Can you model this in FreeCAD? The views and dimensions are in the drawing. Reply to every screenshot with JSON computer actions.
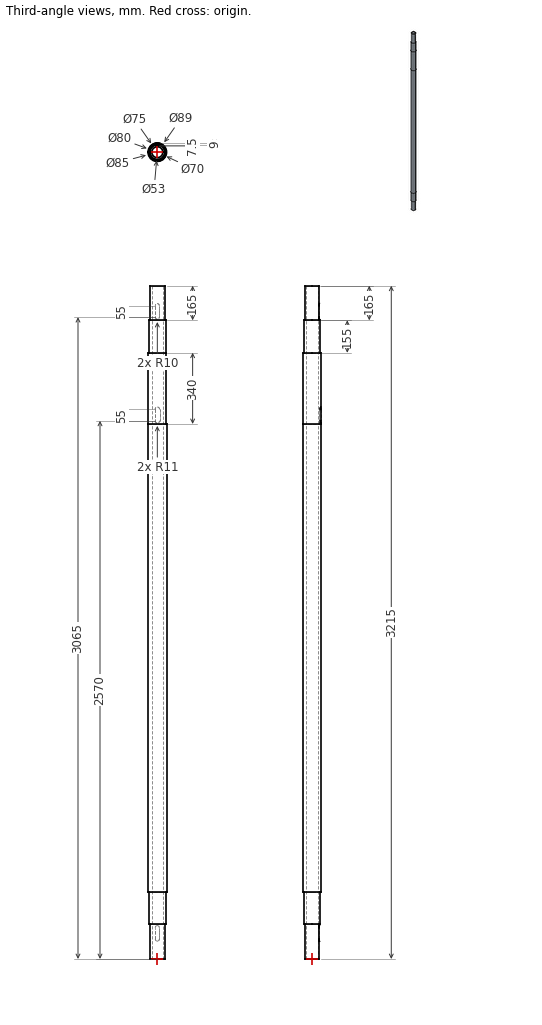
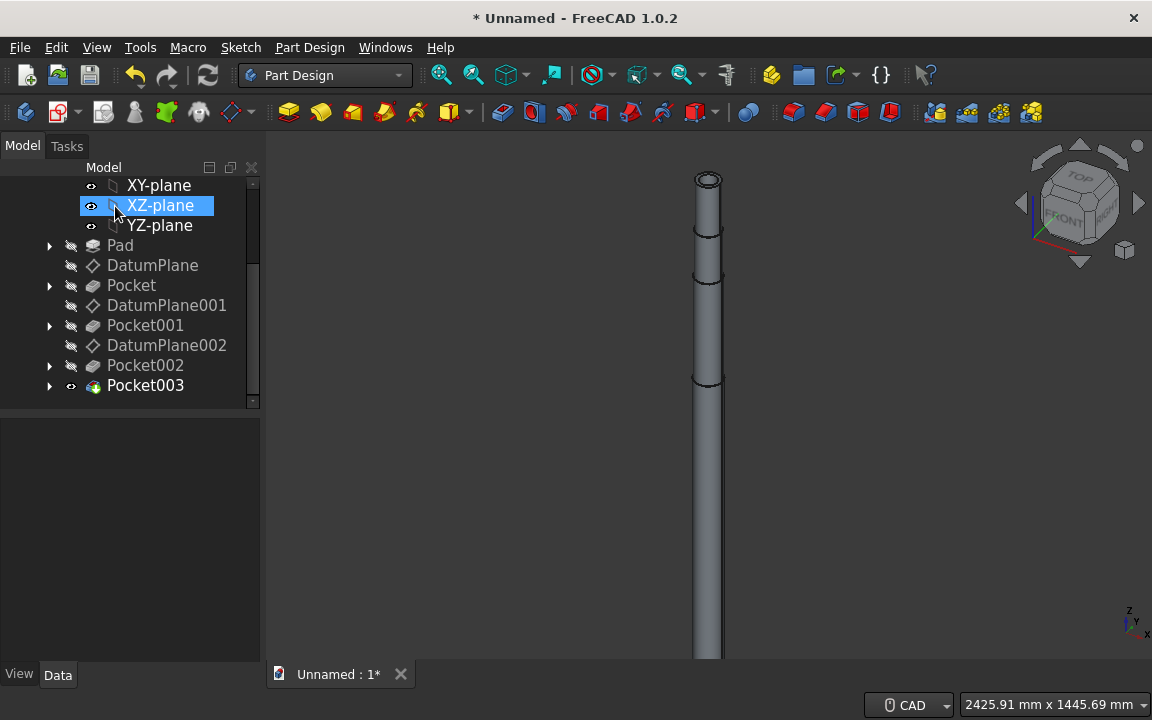
{"action": "left_click", "coordinate": [442, 76]}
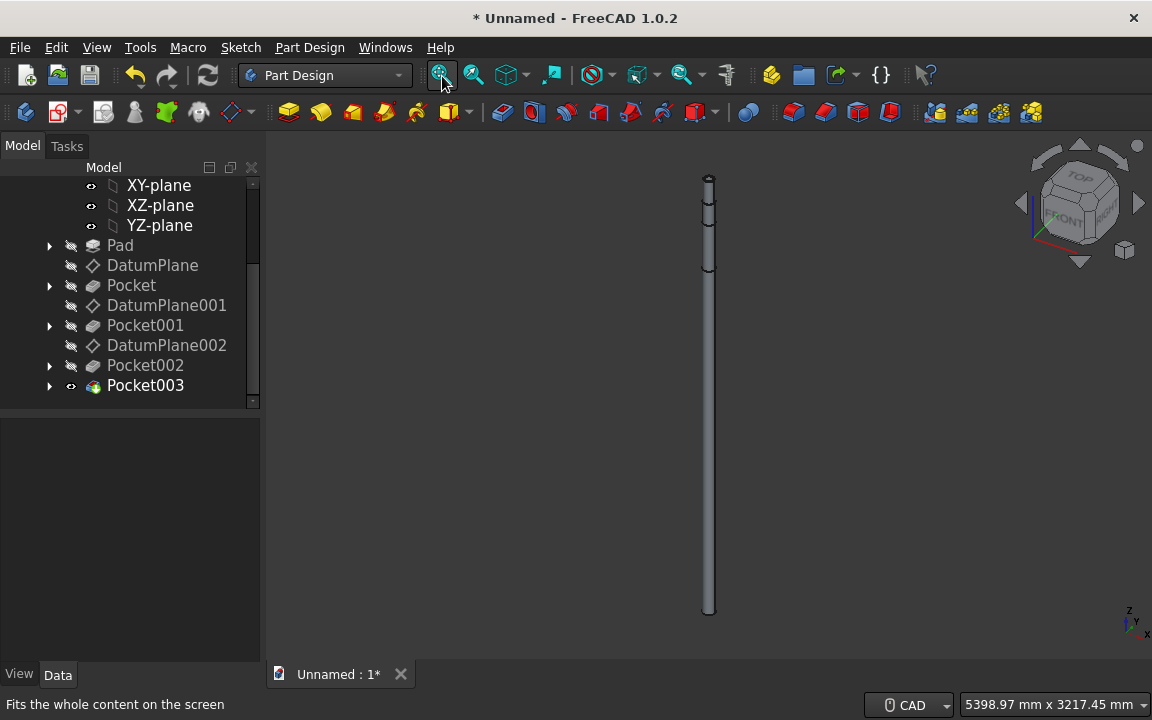
{"action": "scroll", "coordinate": [711, 197], "scroll_direction": "up", "scroll_amount": 15}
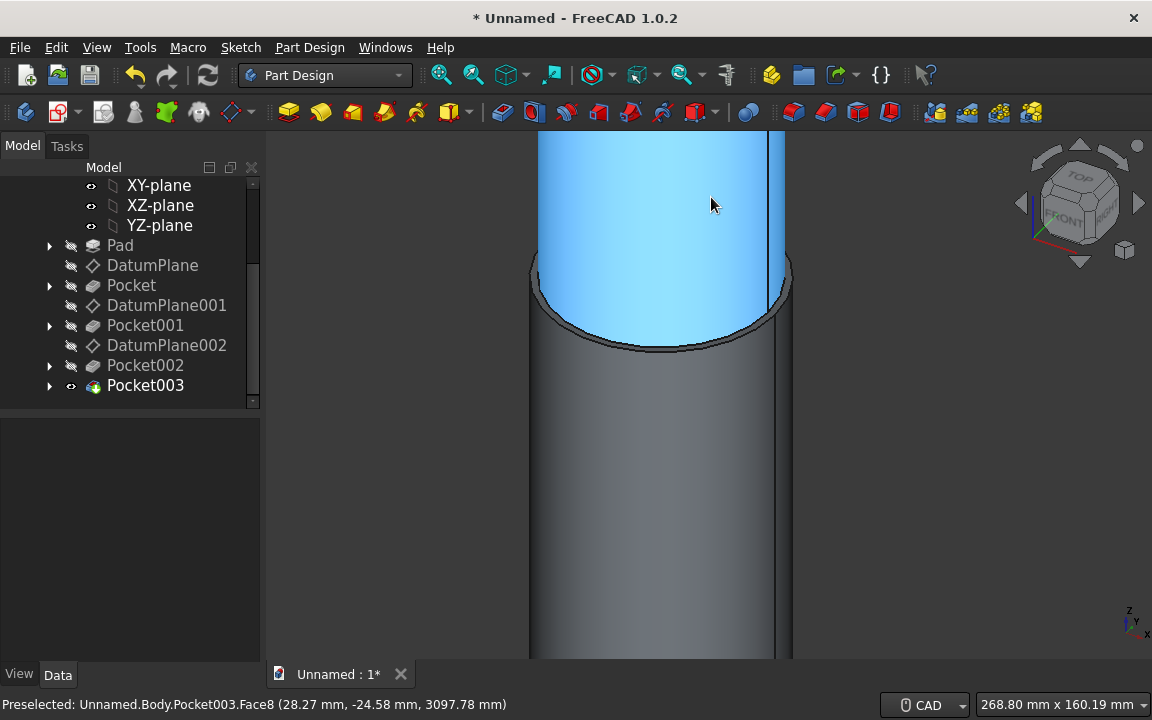
{"action": "scroll", "coordinate": [701, 205], "scroll_direction": "up", "scroll_amount": 8}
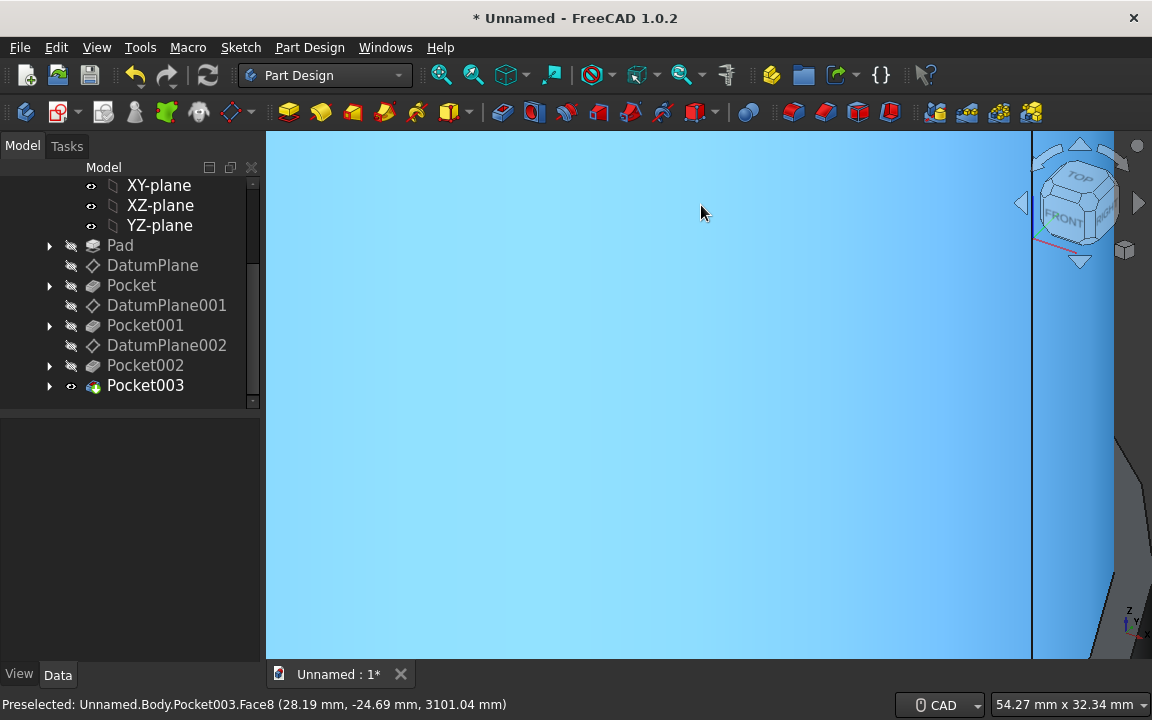
{"action": "left_click", "coordinate": [442, 76]}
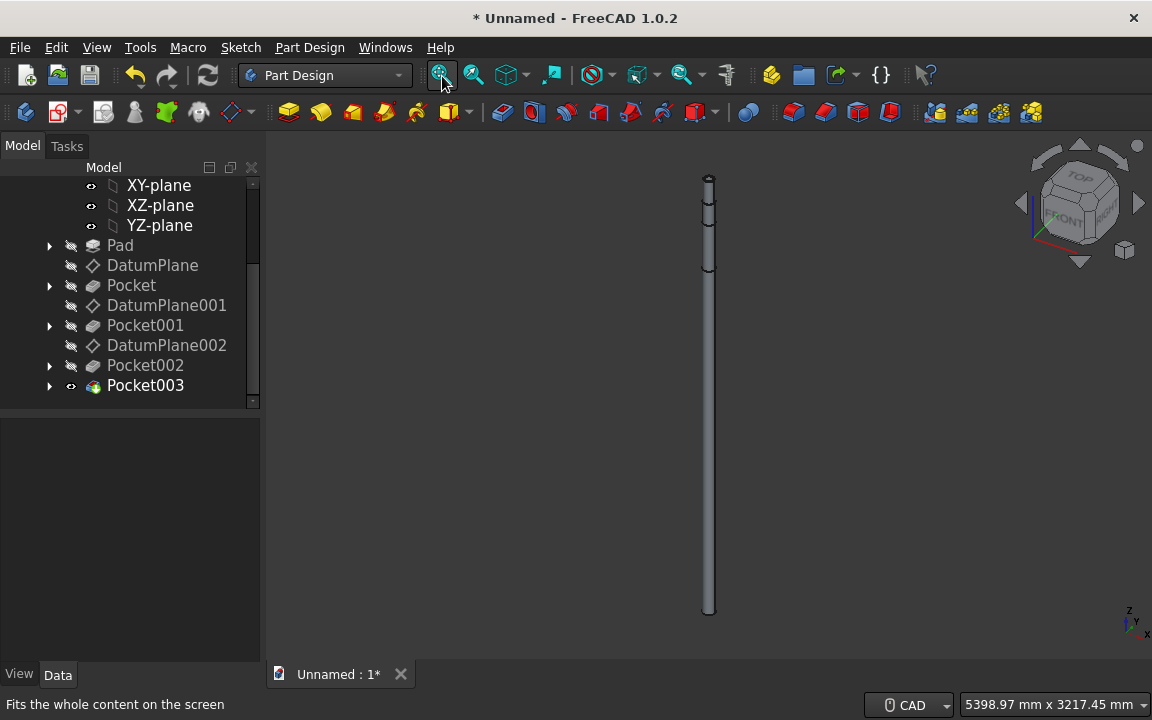
{"action": "key", "text": "0"}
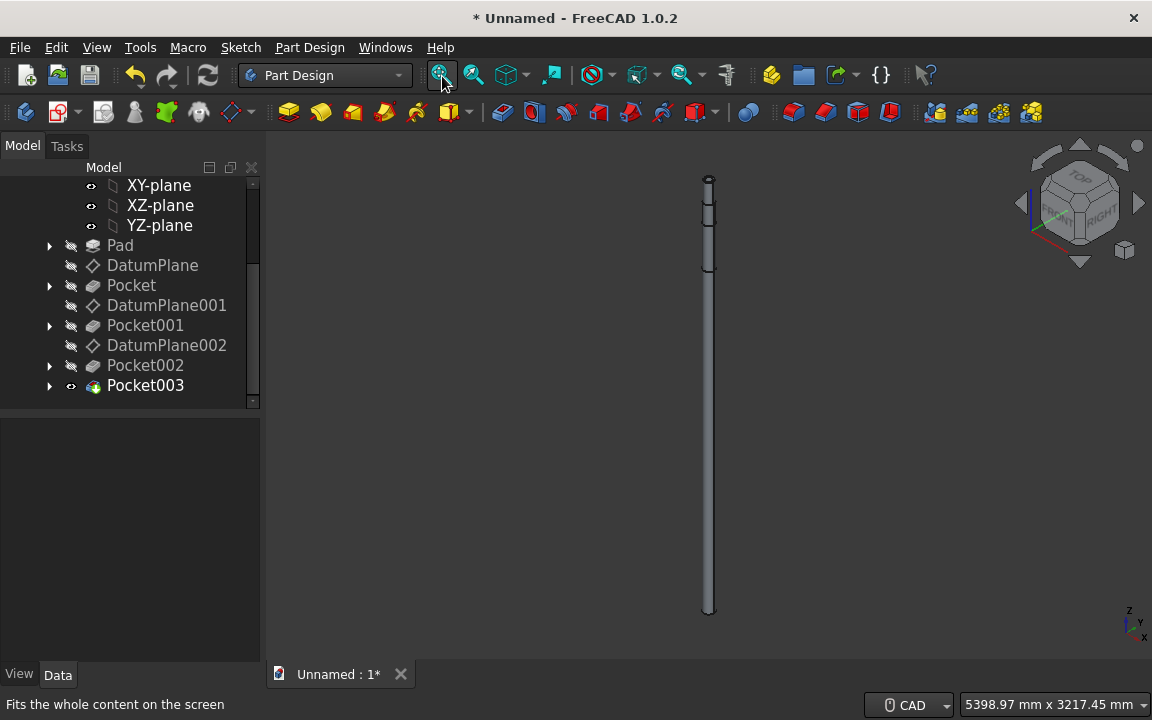
{"action": "scroll", "coordinate": [713, 198], "scroll_direction": "up", "scroll_amount": 15}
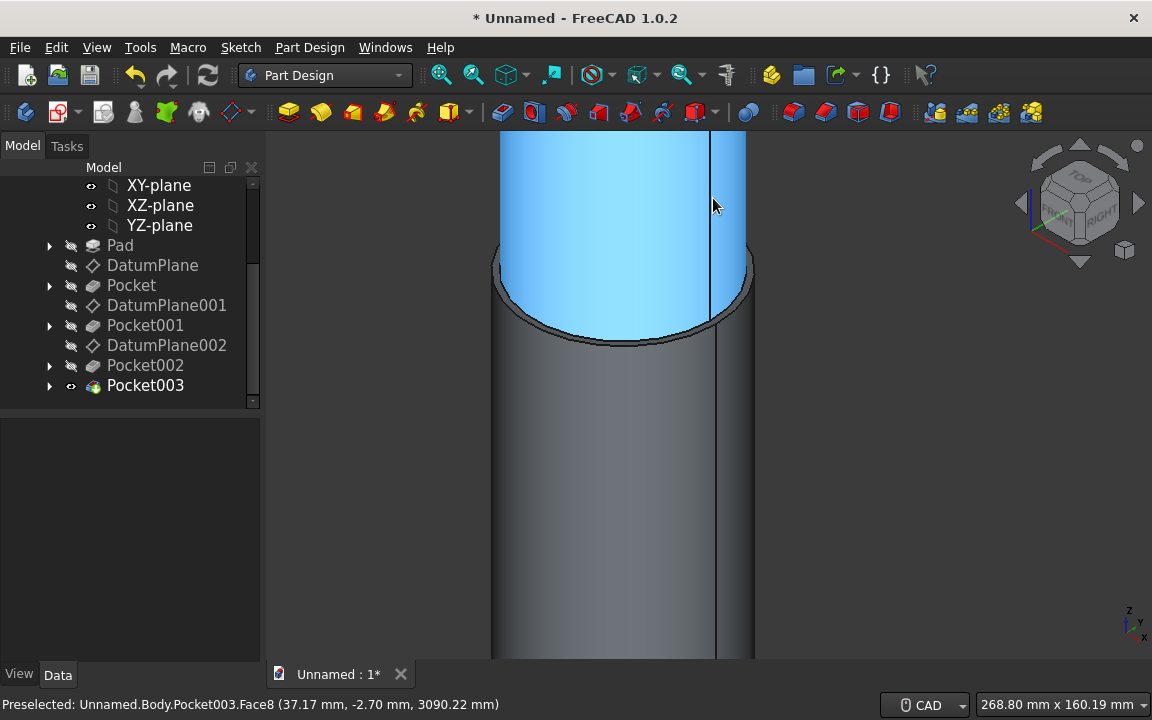
{"action": "scroll", "coordinate": [694, 207], "scroll_direction": "up", "scroll_amount": 8}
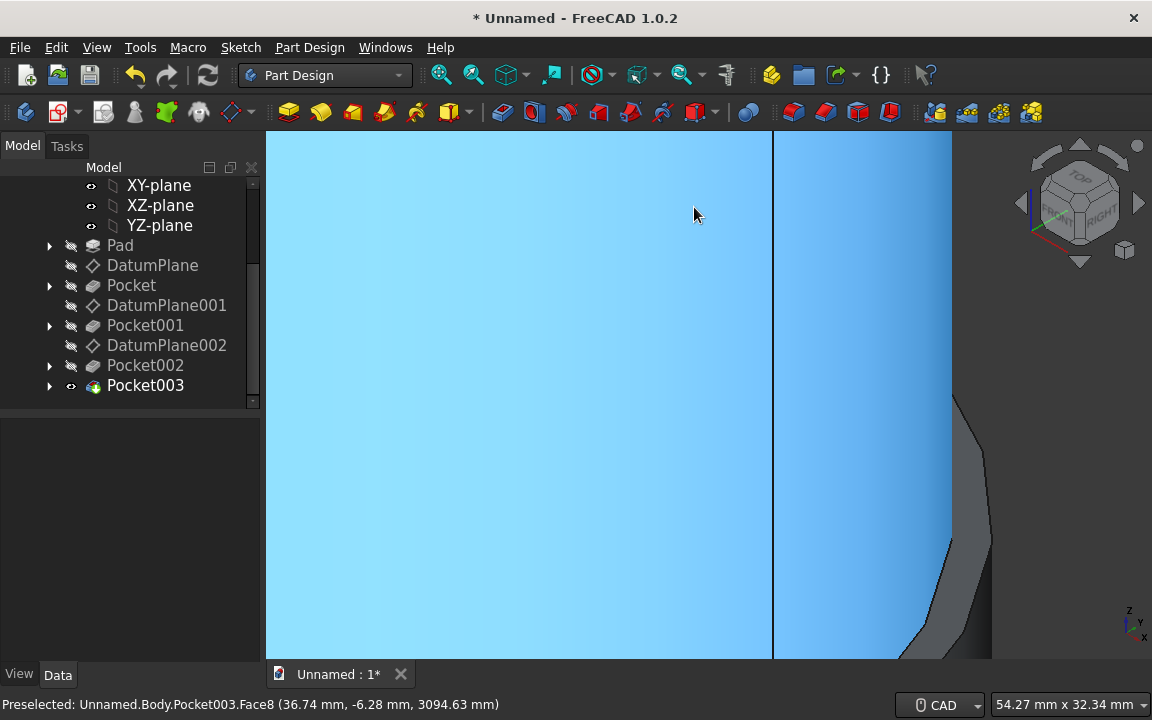
{"action": "left_click", "coordinate": [442, 76]}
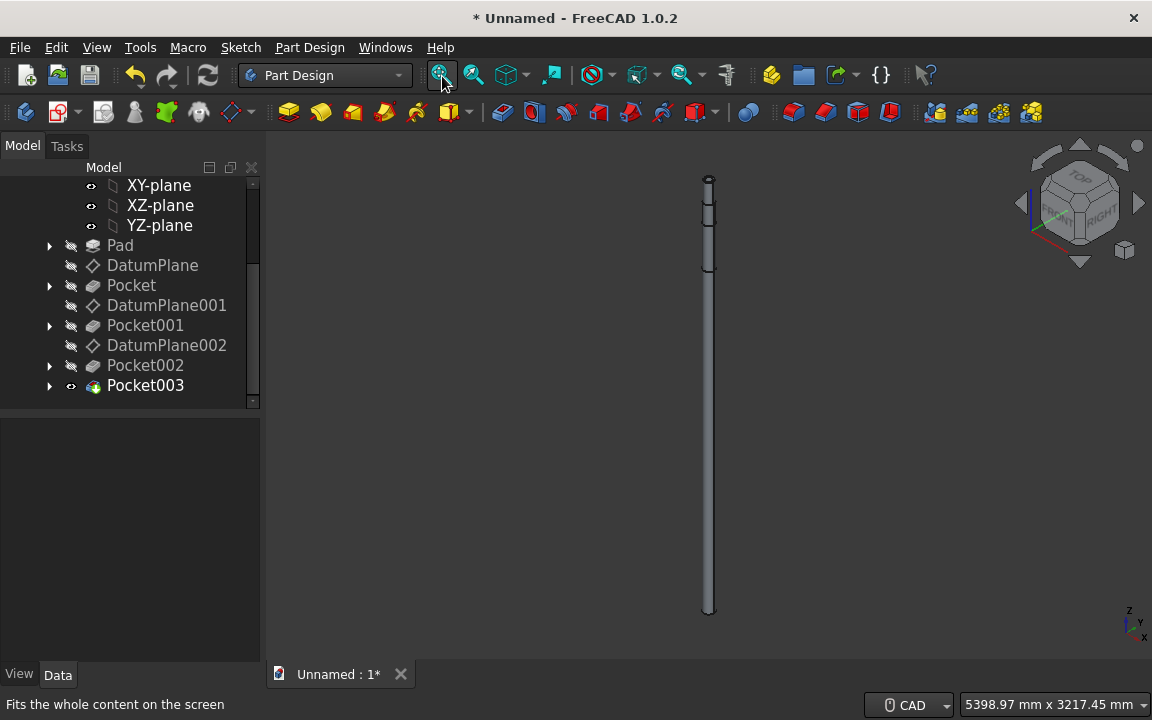
{"action": "key", "text": "2"}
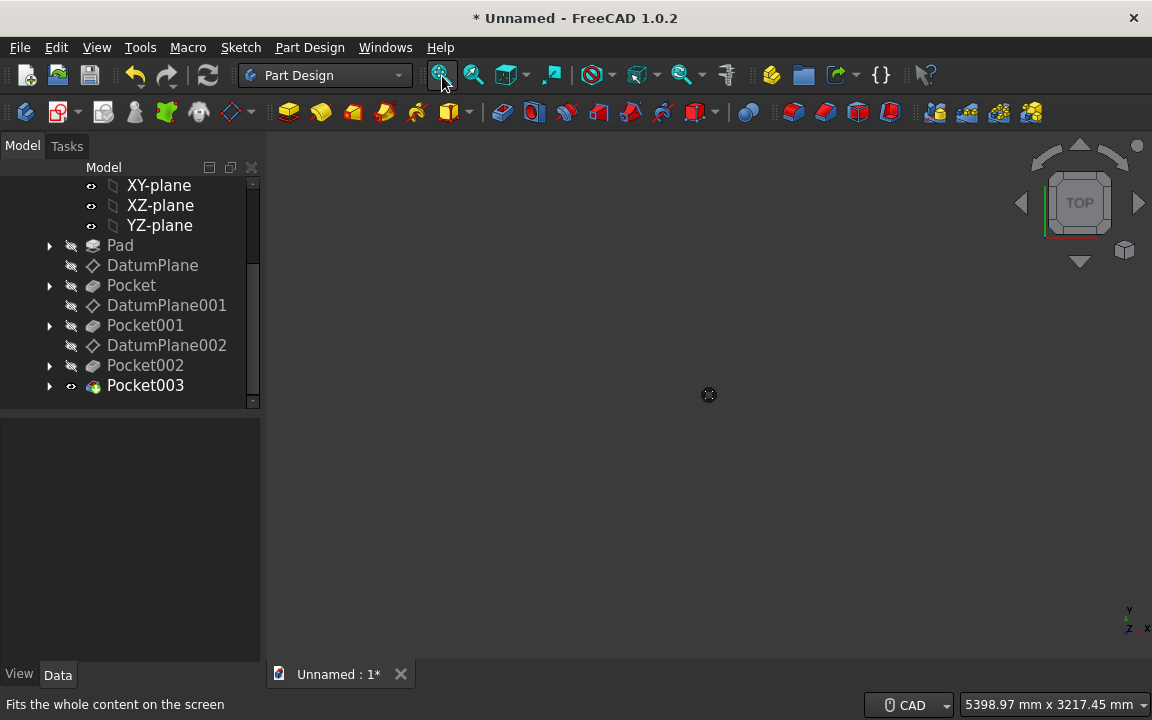
{"action": "left_click", "coordinate": [442, 76]}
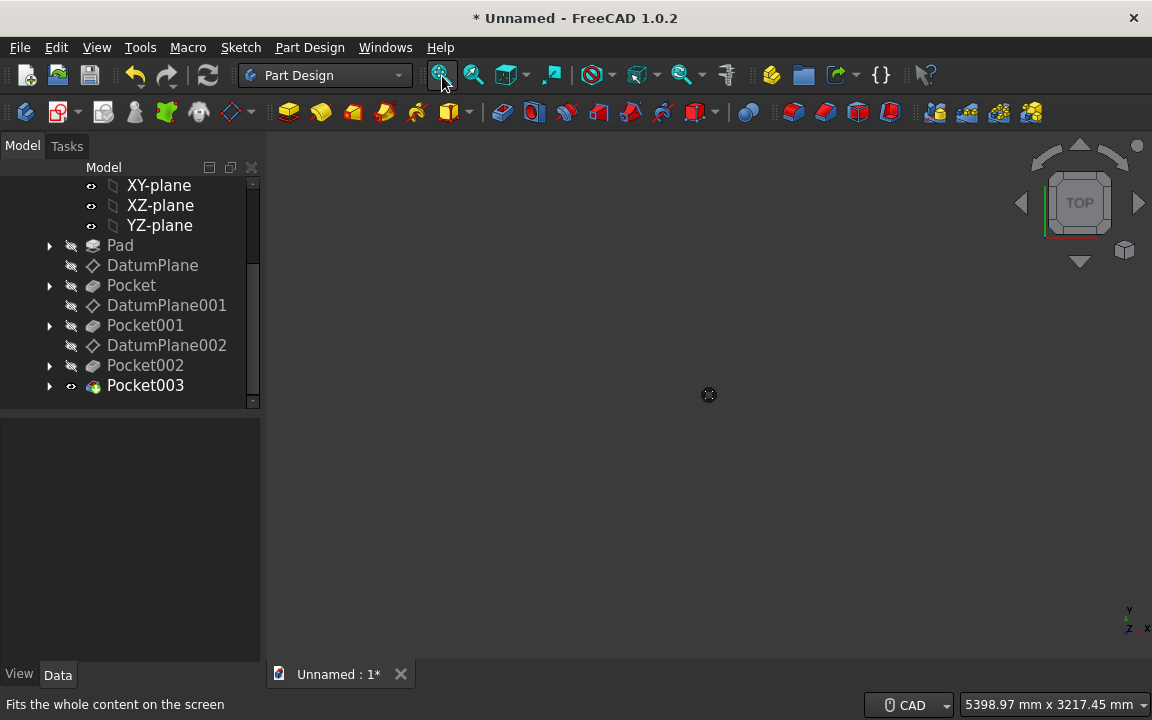
{"action": "scroll", "coordinate": [708, 388], "scroll_direction": "up", "scroll_amount": 15}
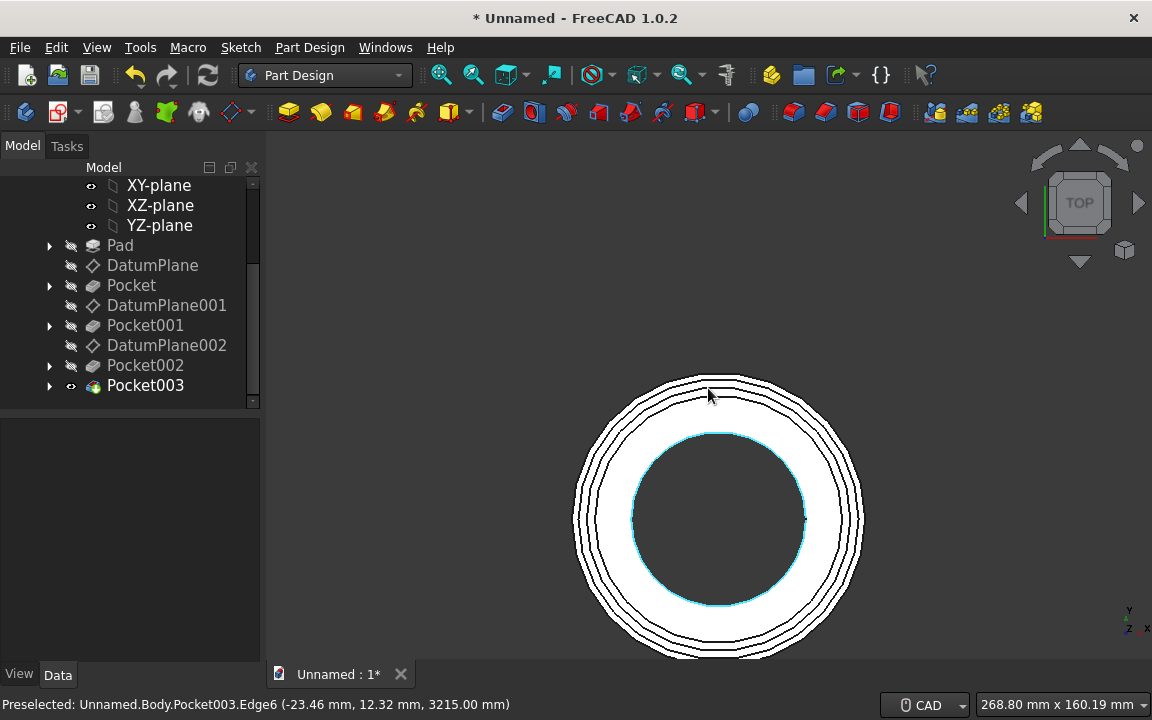
{"action": "scroll", "coordinate": [692, 392], "scroll_direction": "up", "scroll_amount": 8}